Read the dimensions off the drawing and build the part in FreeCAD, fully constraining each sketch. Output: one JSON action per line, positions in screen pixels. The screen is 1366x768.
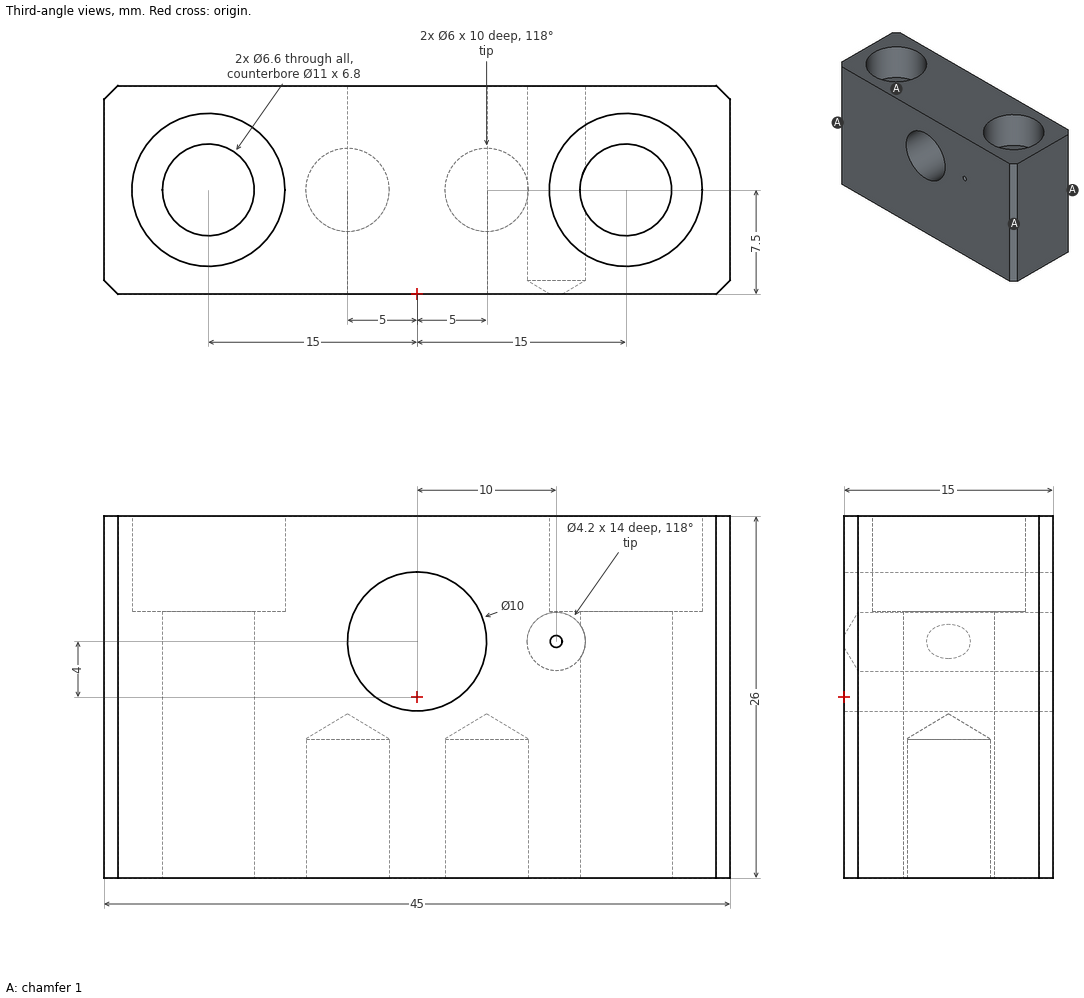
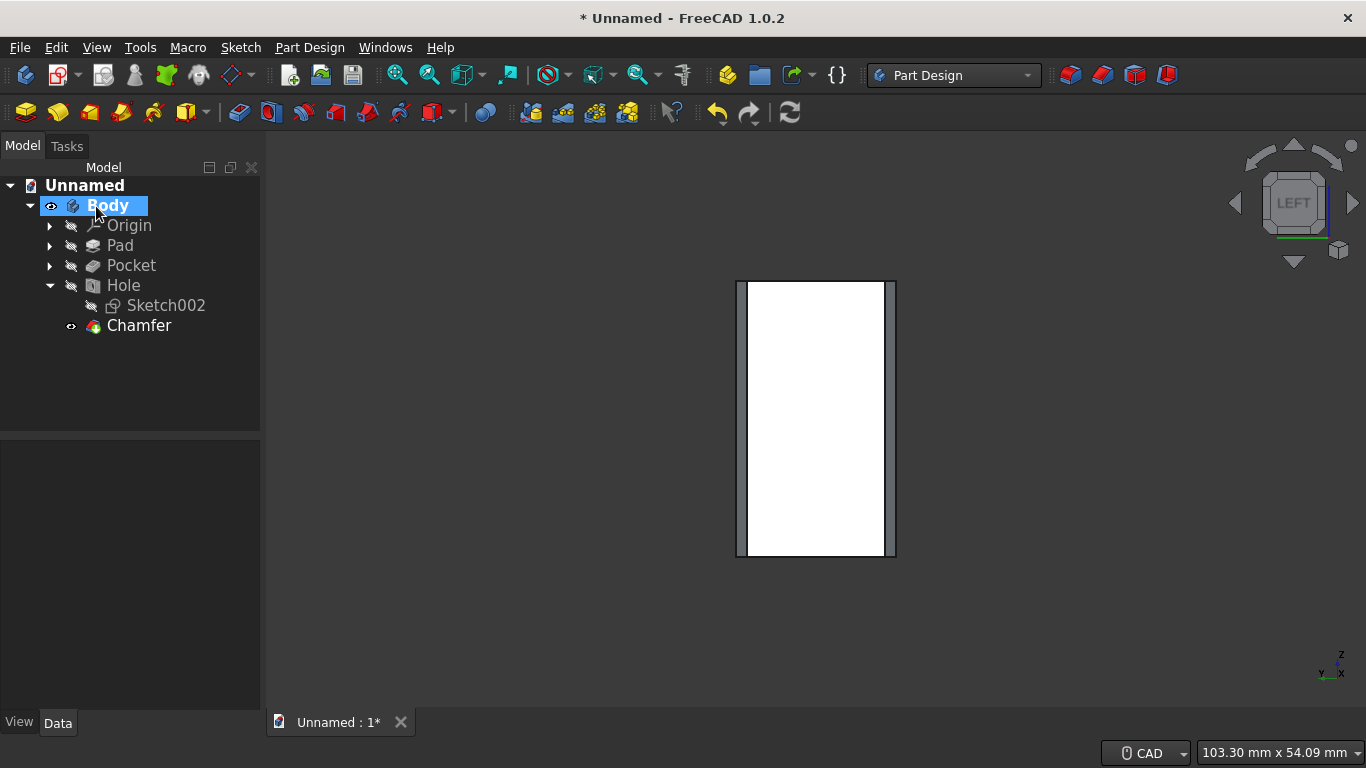
{"action": "key", "text": "0"}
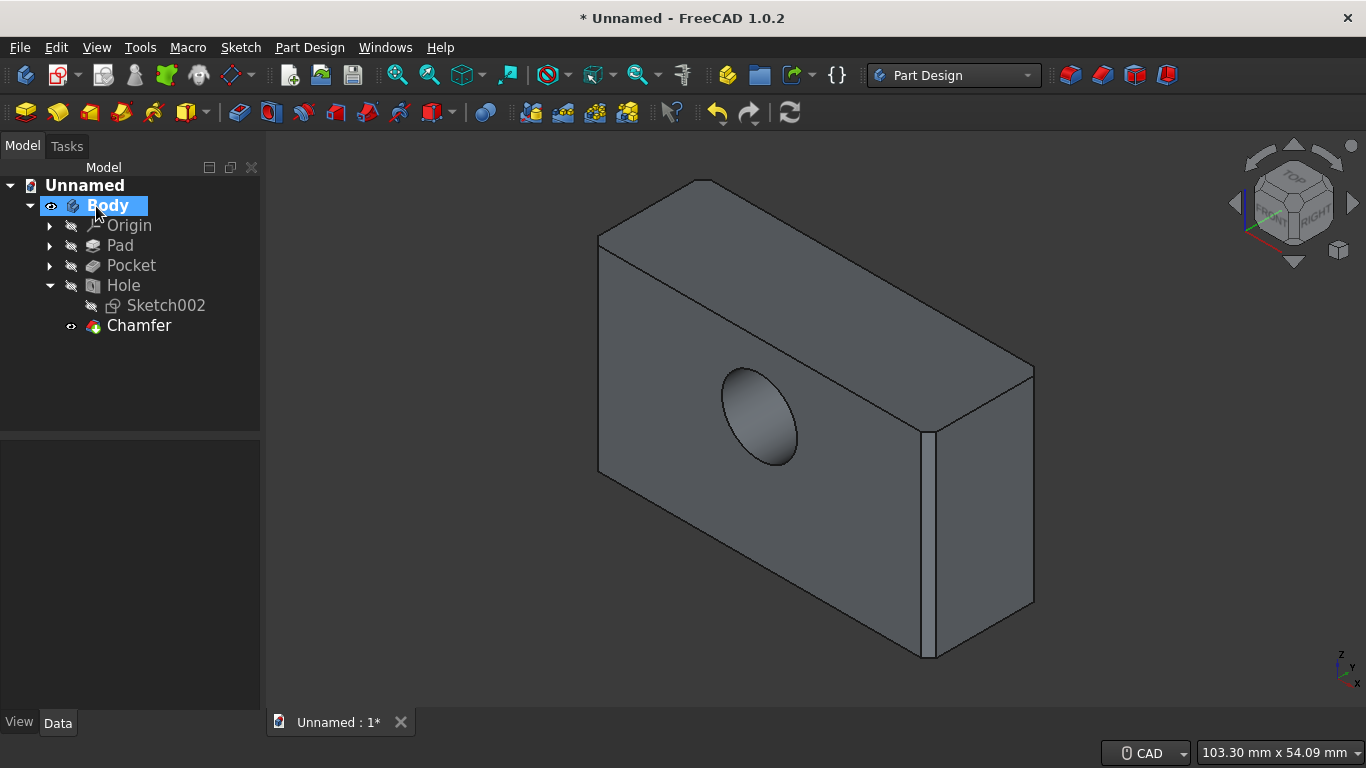
{"action": "left_click", "coordinate": [913, 361]}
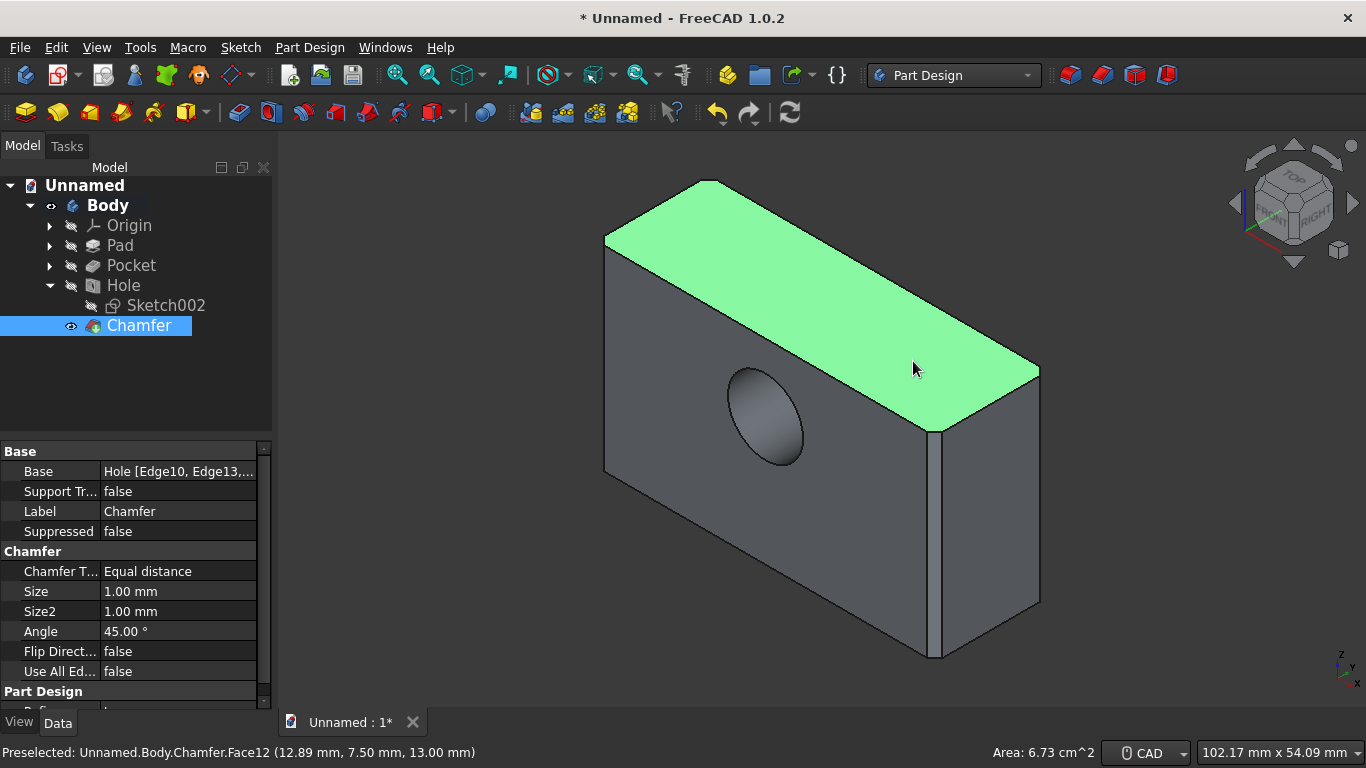
{"action": "left_click", "coordinate": [58, 76]}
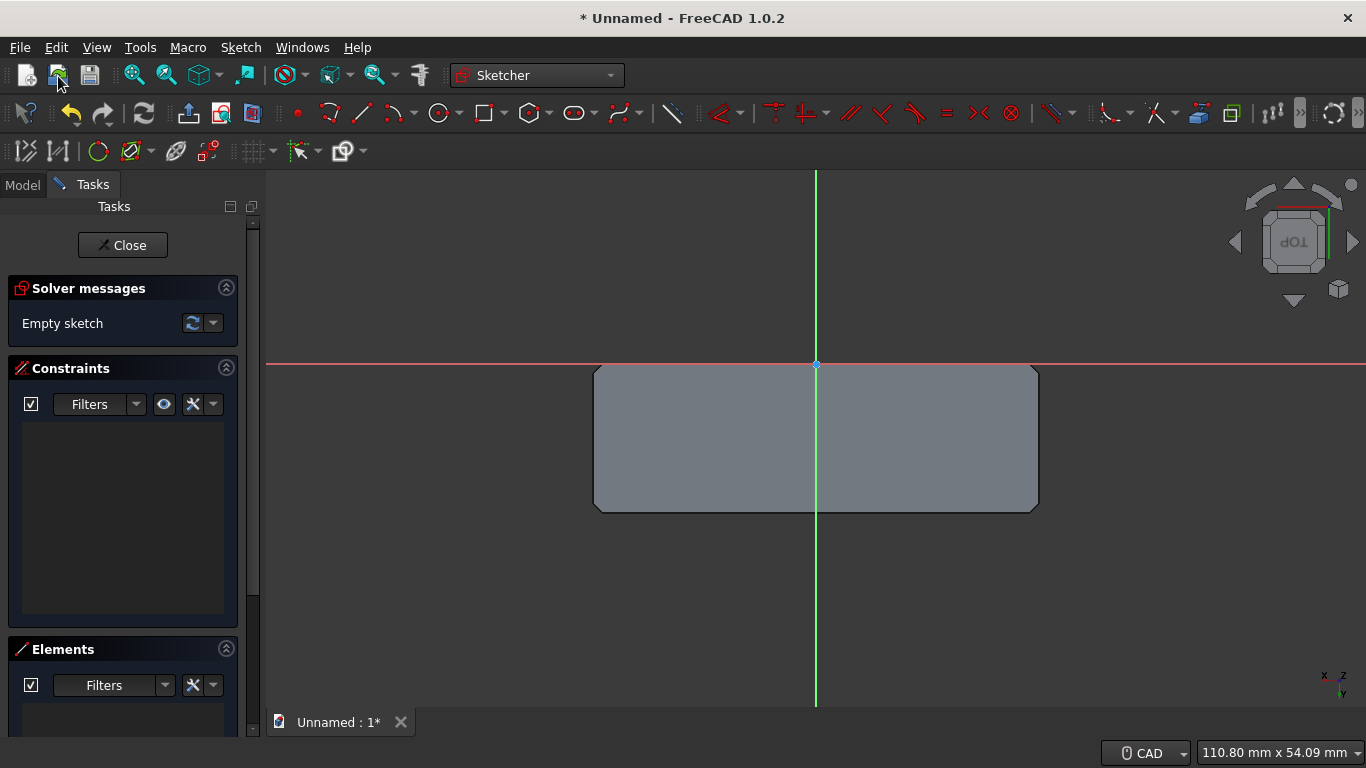
{"action": "scroll", "coordinate": [899, 392], "scroll_direction": "up", "scroll_amount": 3}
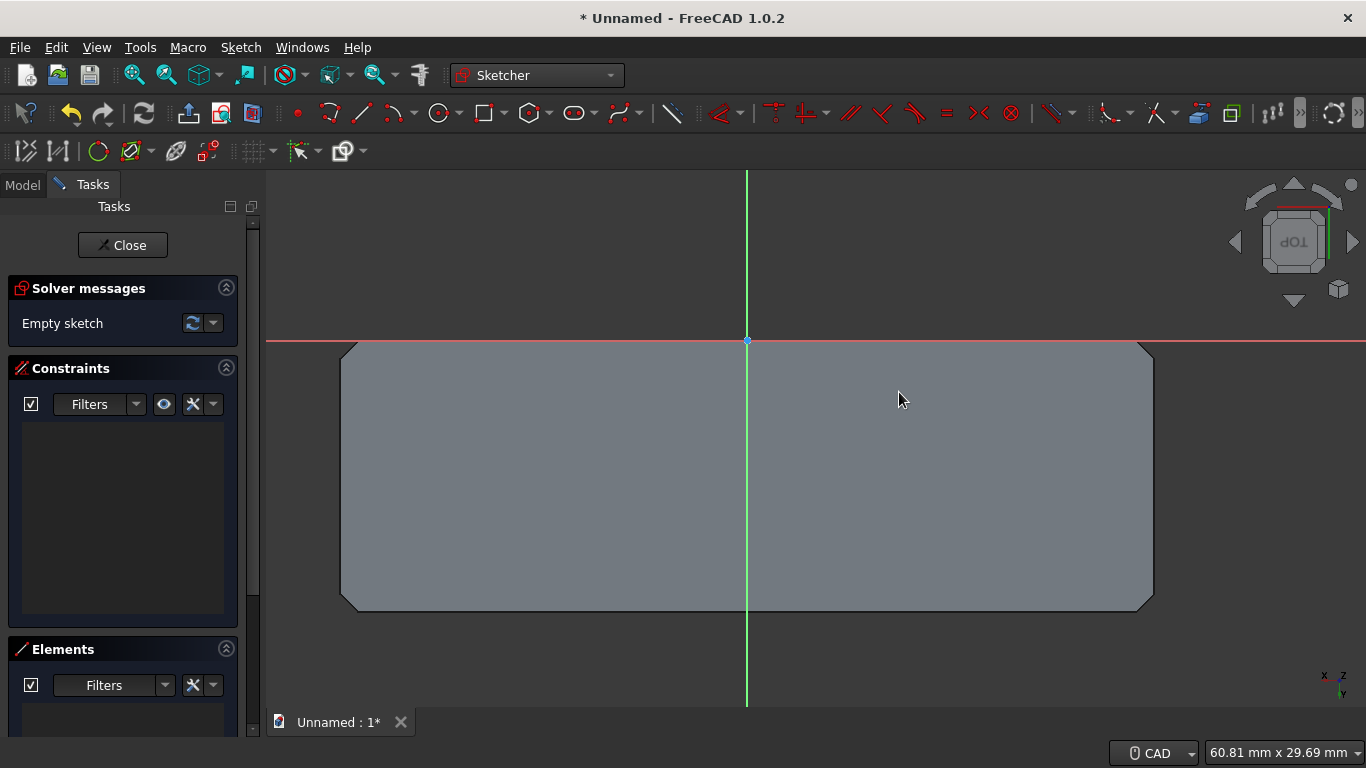
{"action": "left_click", "coordinate": [440, 114]}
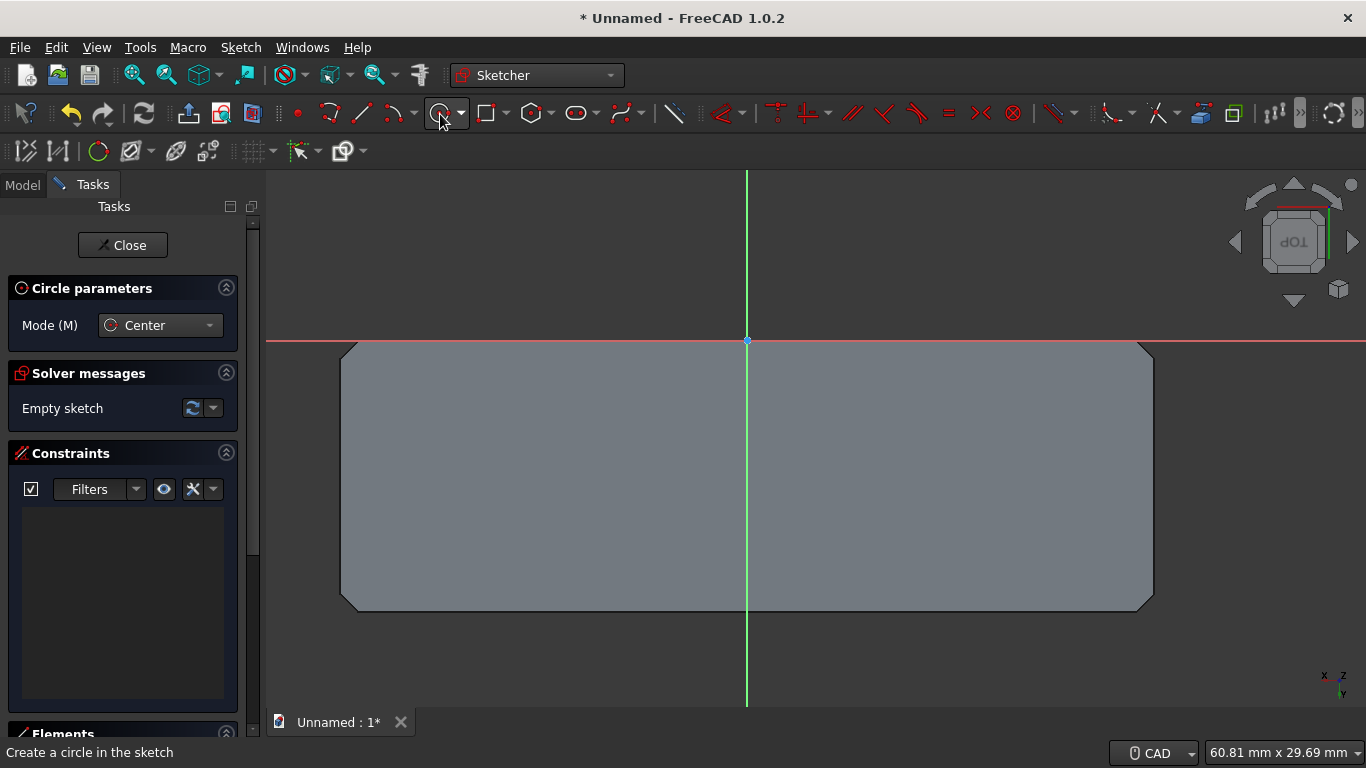
{"action": "left_click", "coordinate": [1019, 476]}
{"action": "left_click", "coordinate": [1061, 434]}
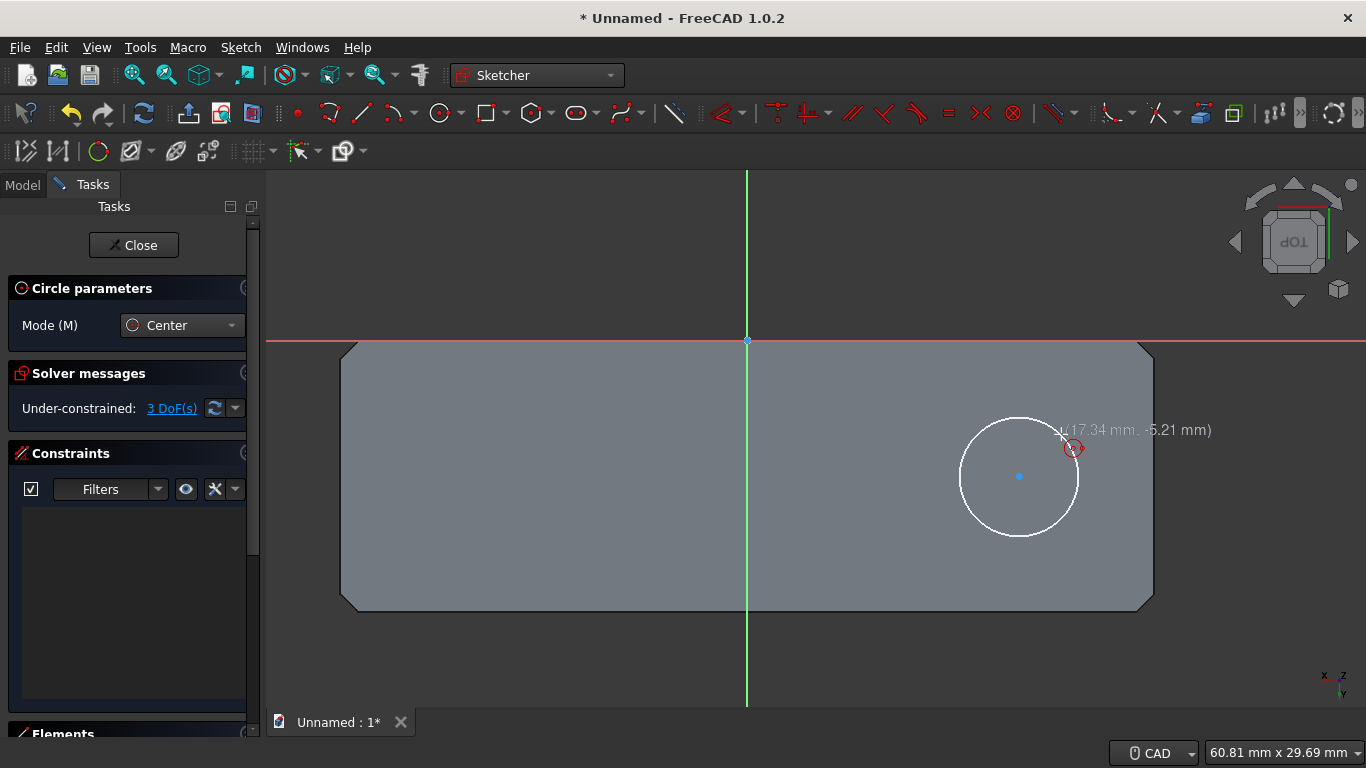
{"action": "left_click", "coordinate": [476, 476]}
{"action": "left_click", "coordinate": [518, 434]}
{"action": "key", "text": "Escape"}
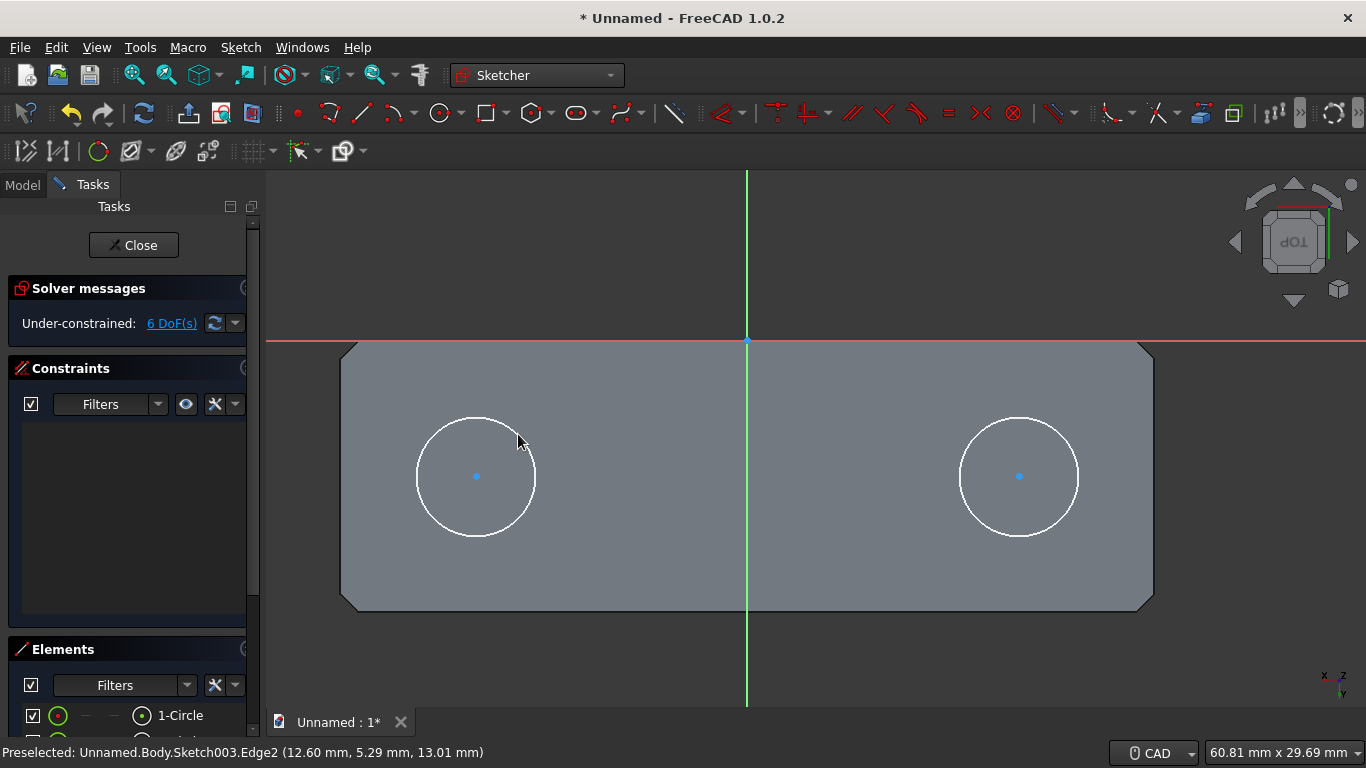
{"action": "left_click", "coordinate": [1061, 435]}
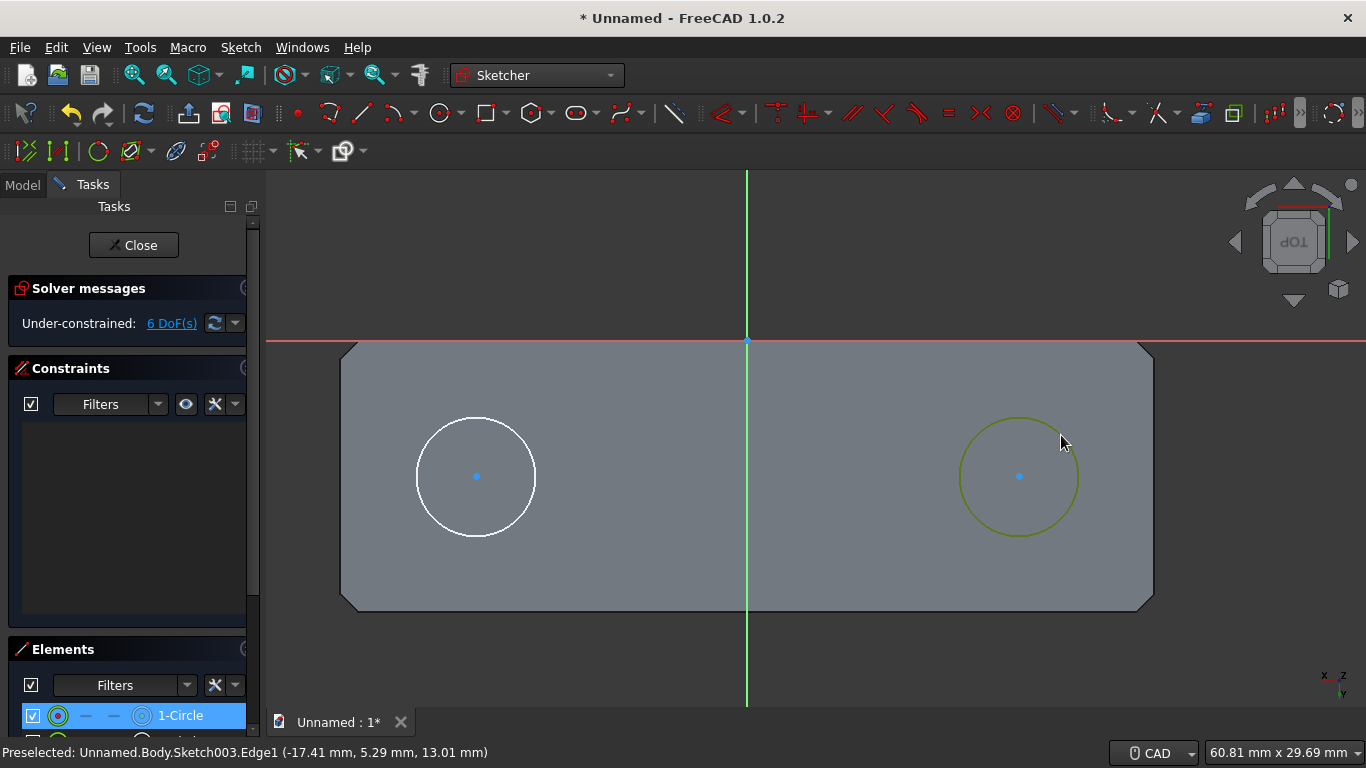
{"action": "left_click", "coordinate": [518, 435]}